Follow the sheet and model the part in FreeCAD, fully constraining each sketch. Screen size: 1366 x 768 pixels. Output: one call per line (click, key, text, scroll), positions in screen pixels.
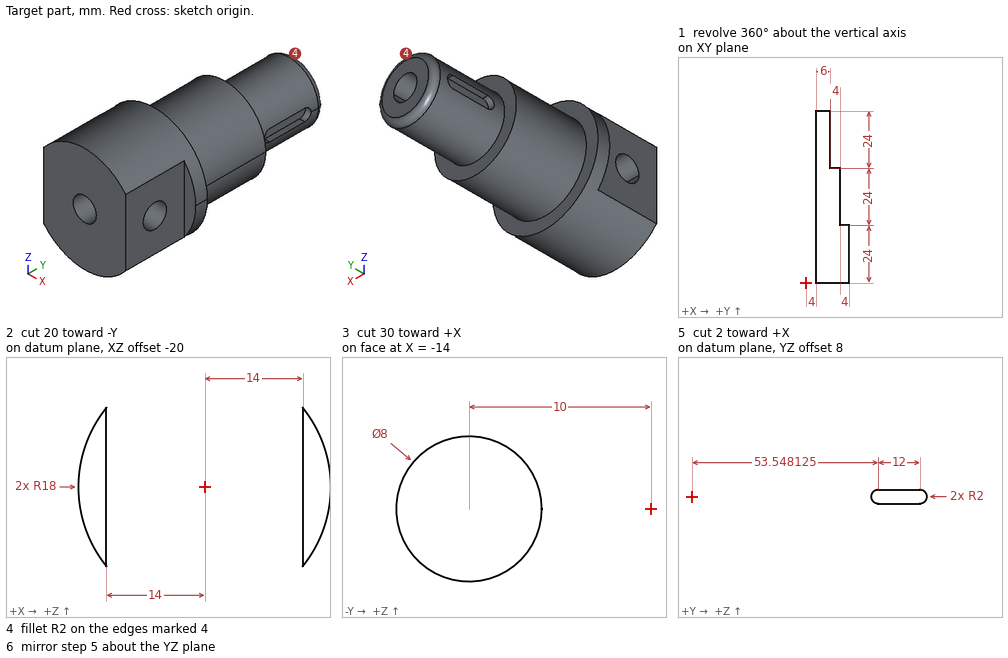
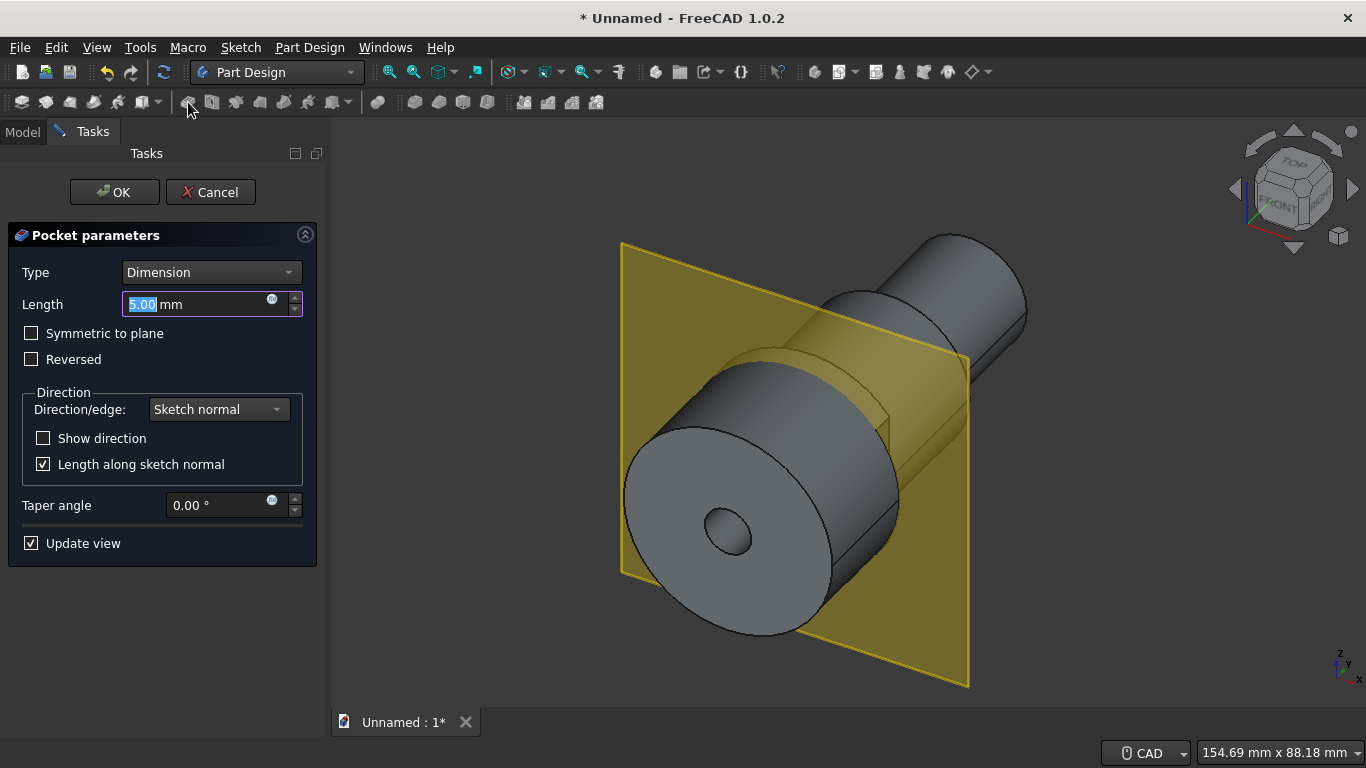
text(20)
key(Tab)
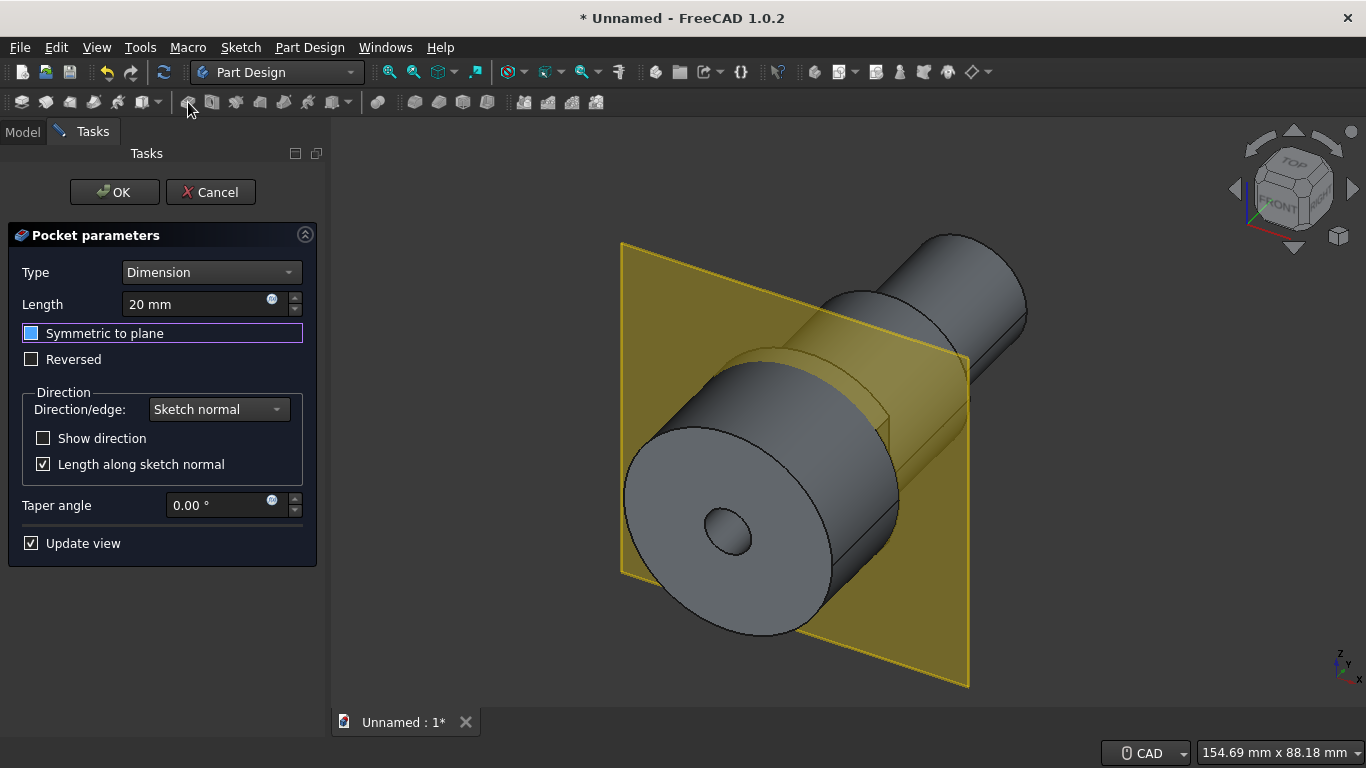
click(30, 359)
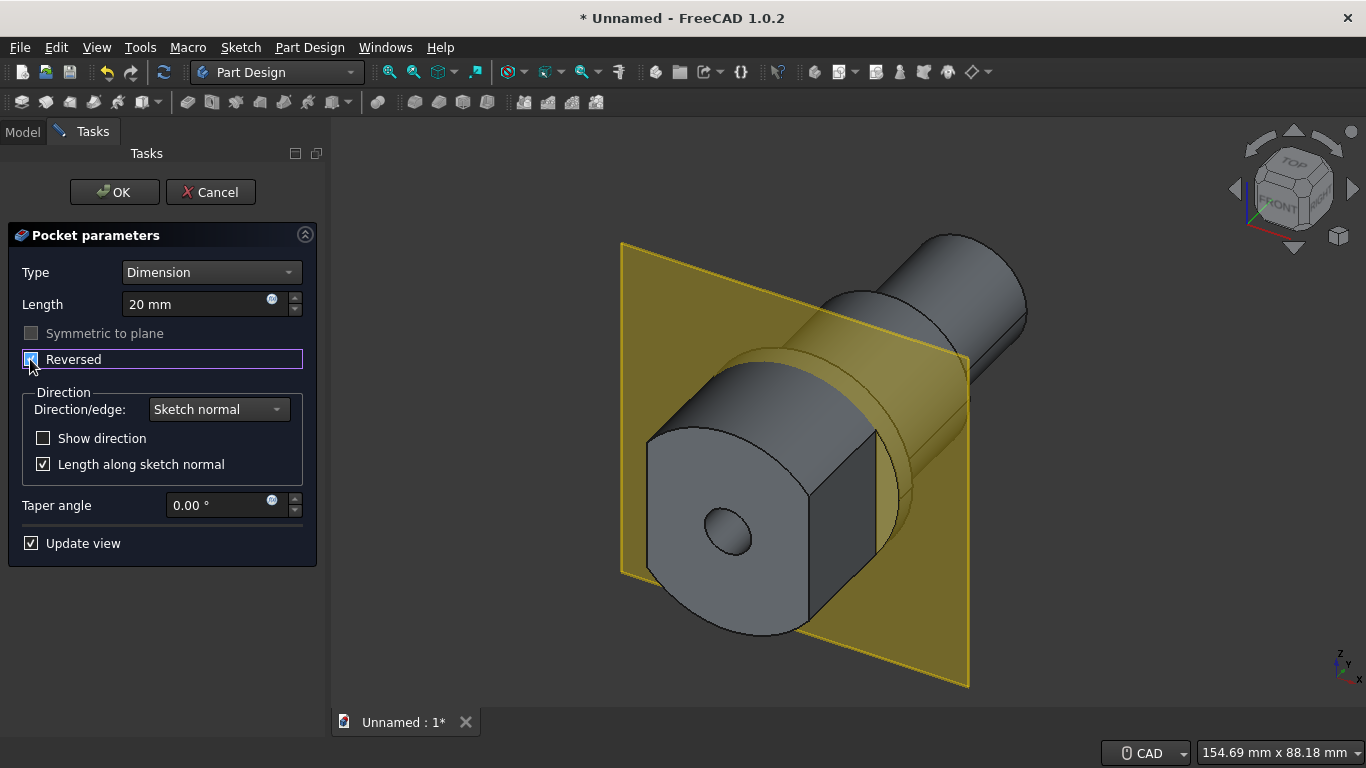
click(115, 192)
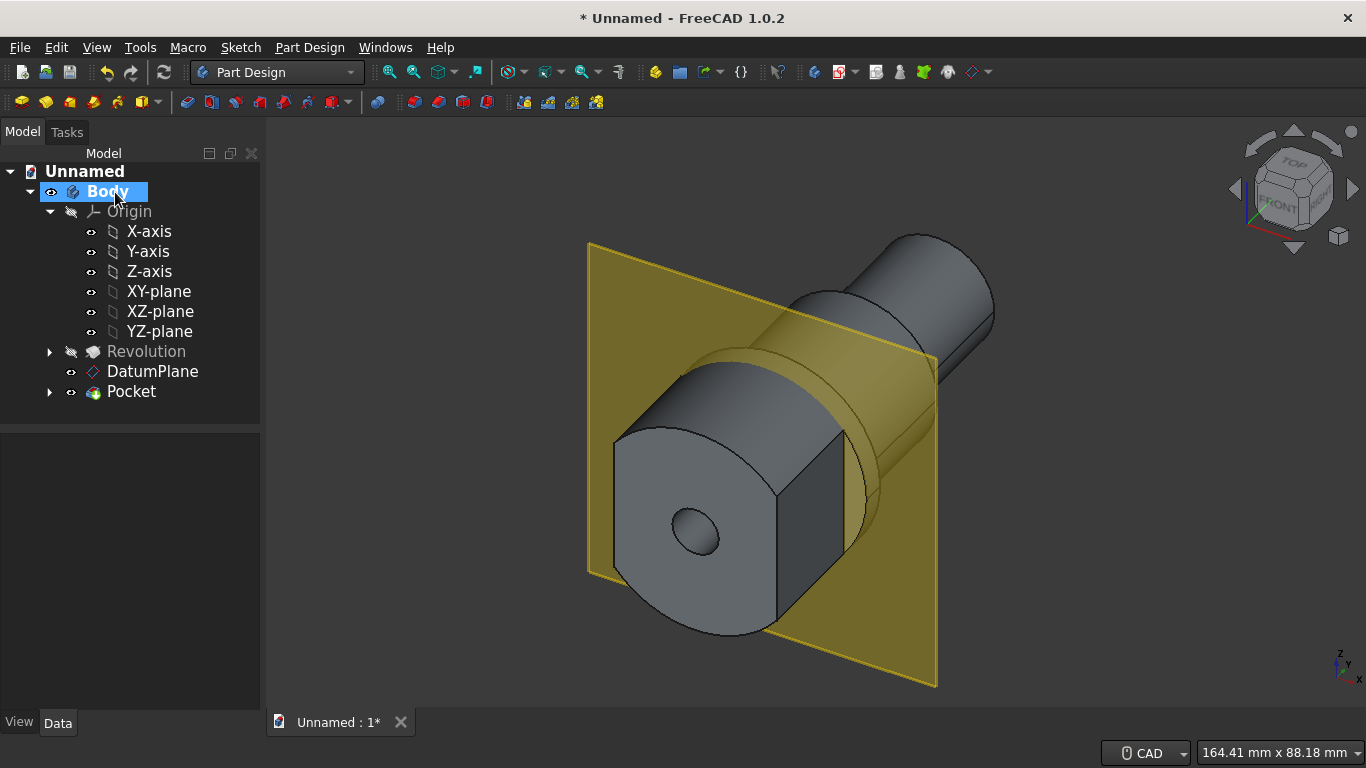
click(116, 372)
key(space)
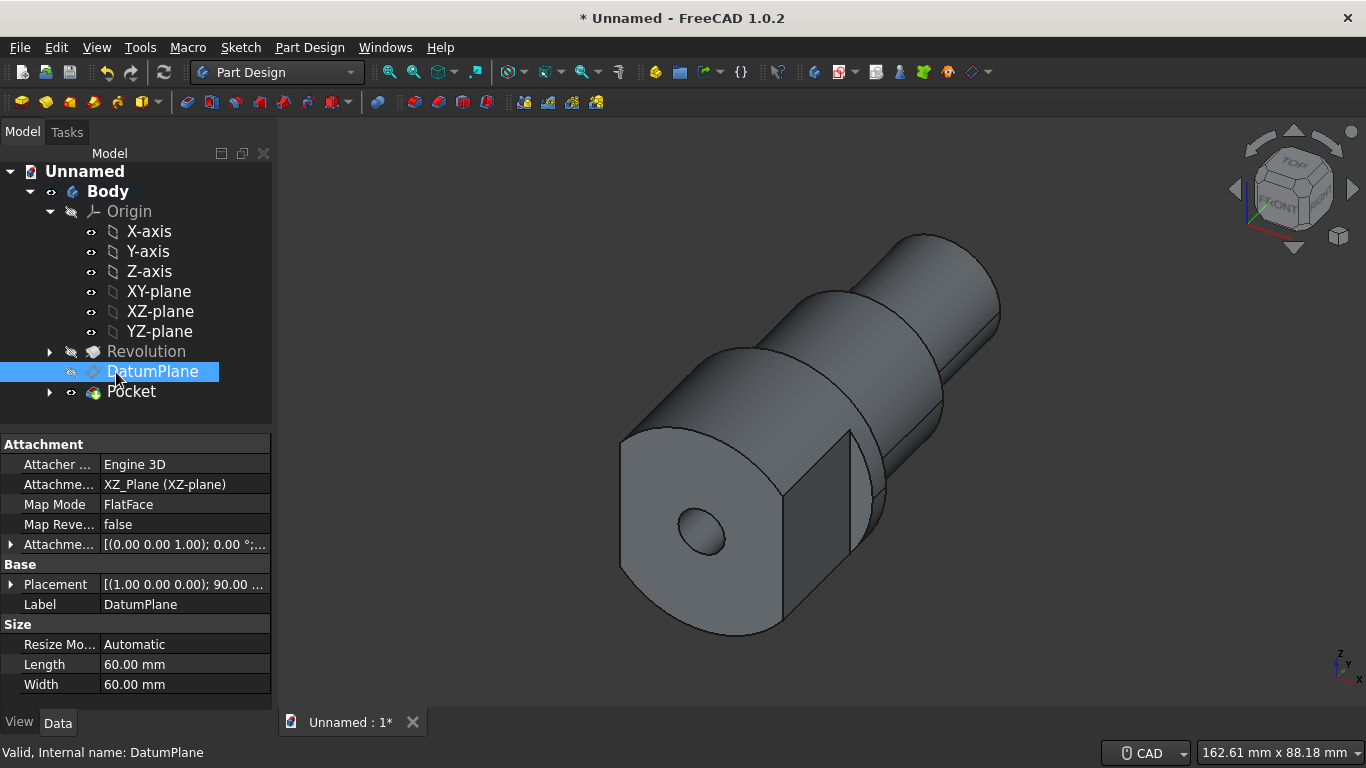
key(6)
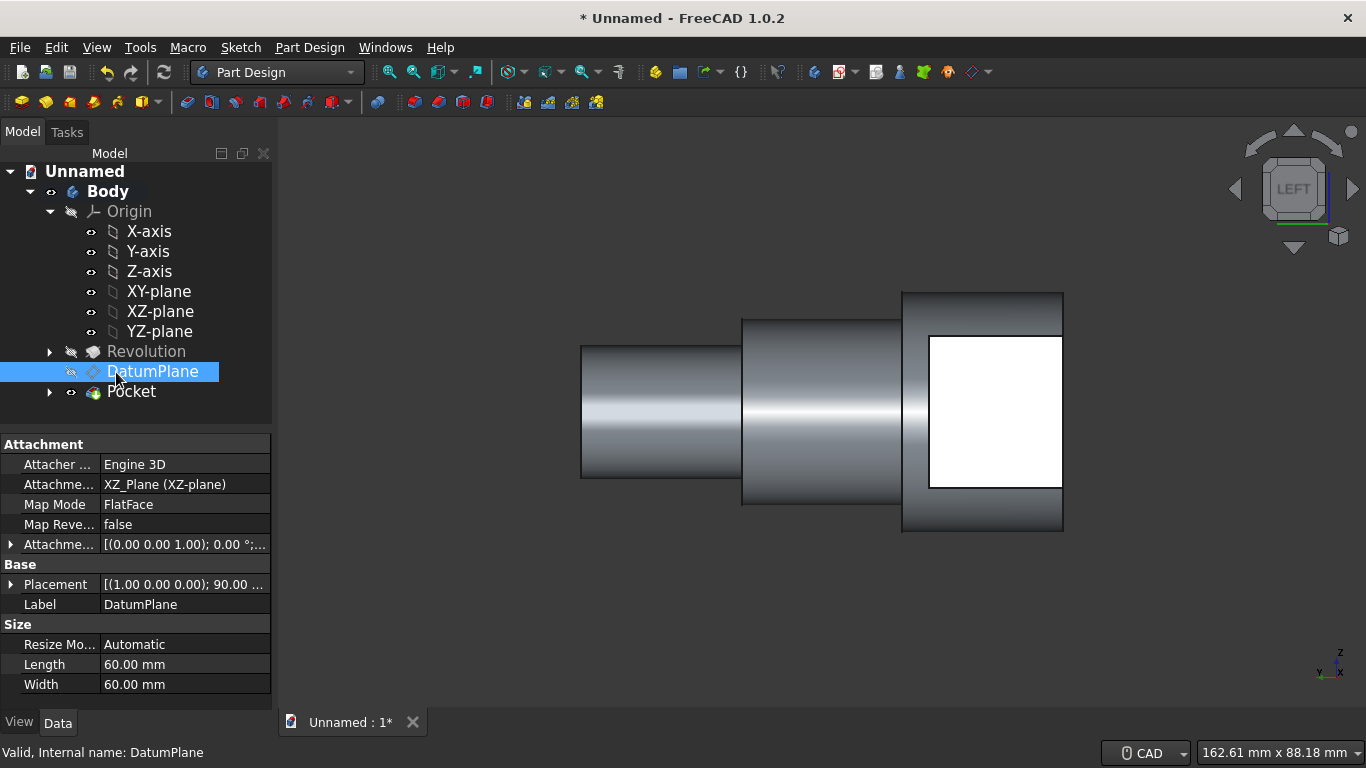
click(390, 72)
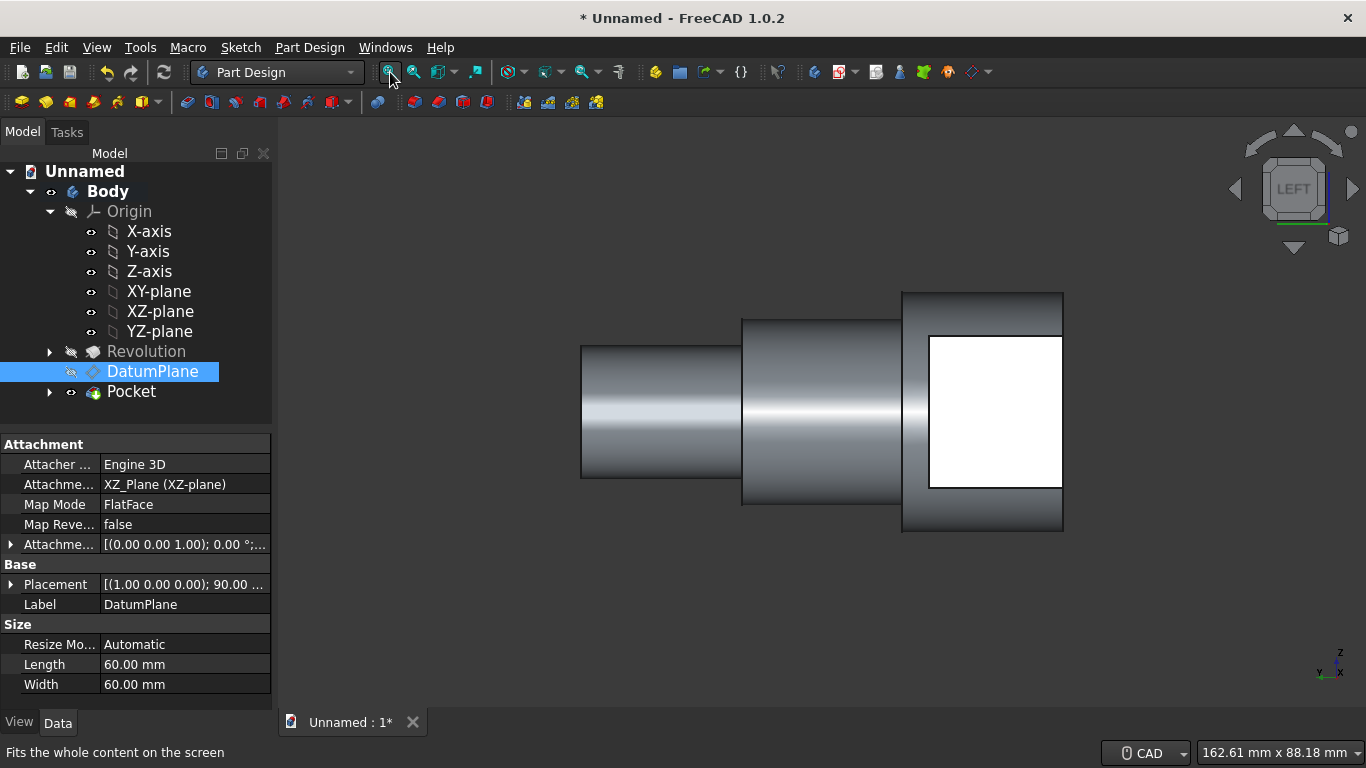
click(996, 411)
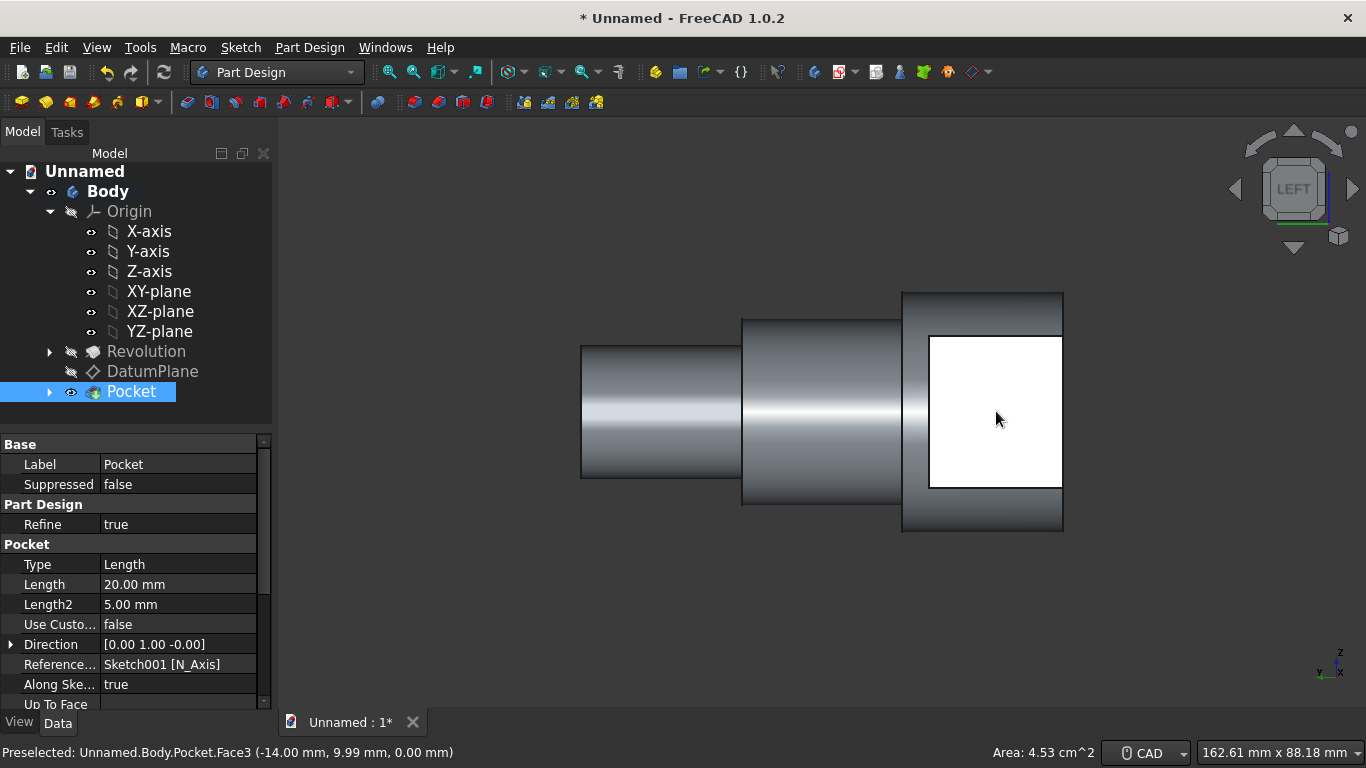
click(840, 72)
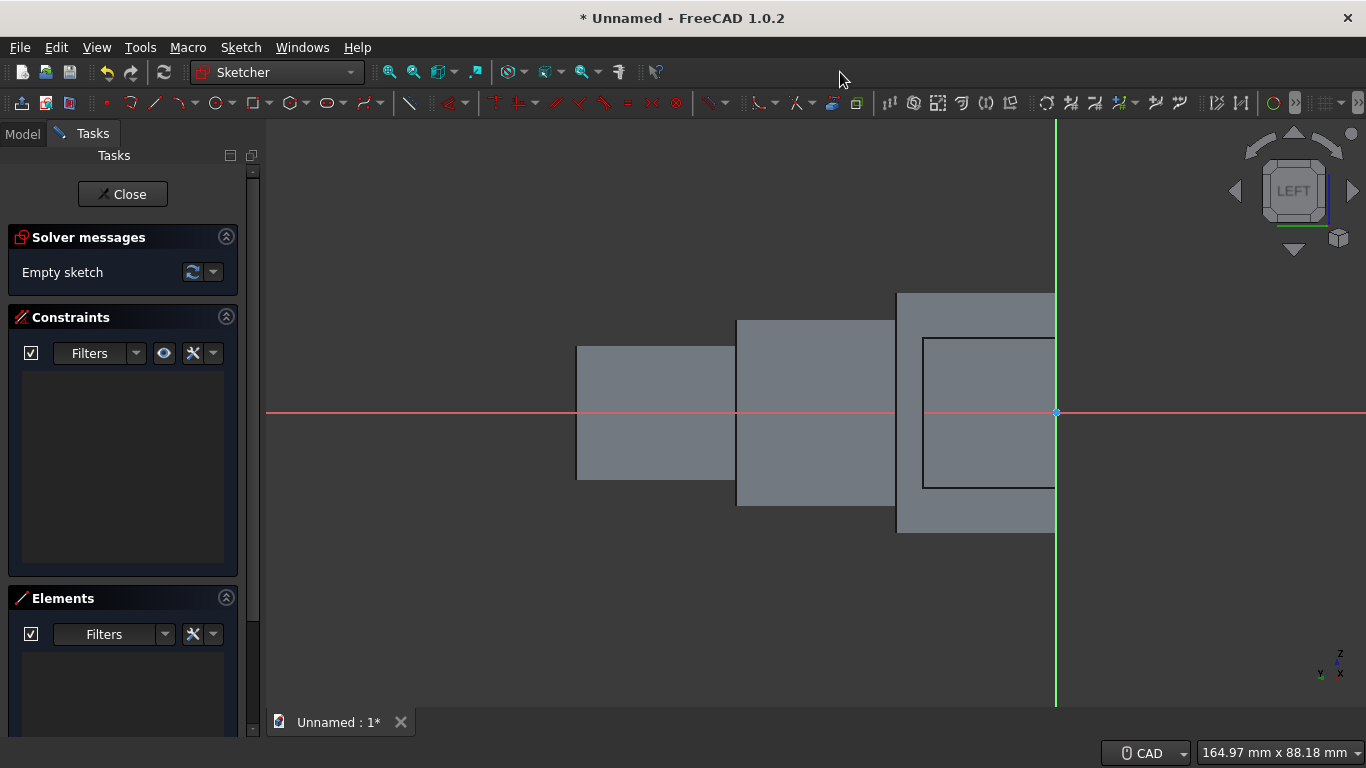
click(70, 104)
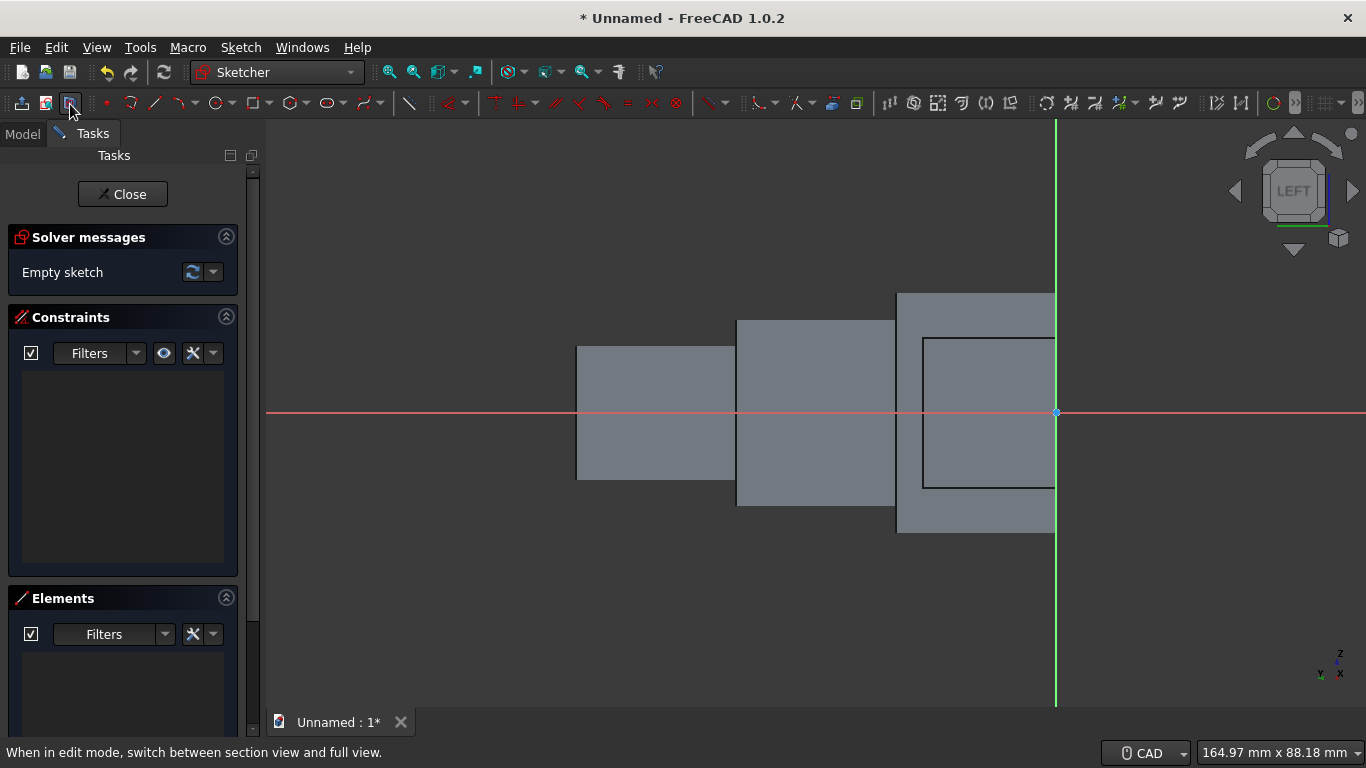
scroll(1050, 413, up, 10)